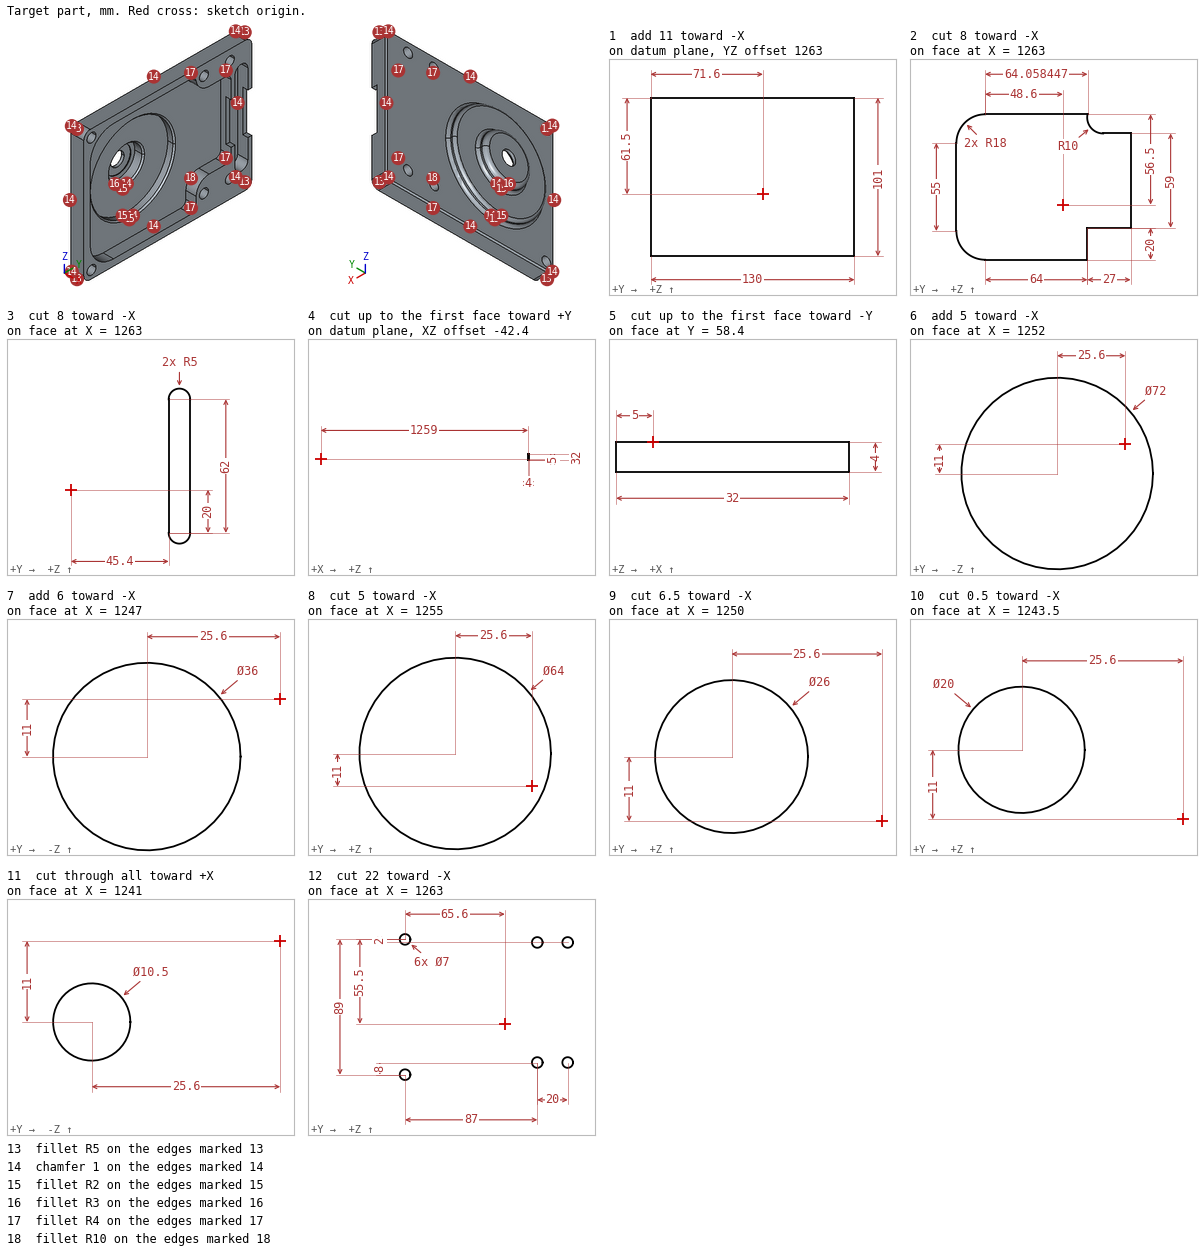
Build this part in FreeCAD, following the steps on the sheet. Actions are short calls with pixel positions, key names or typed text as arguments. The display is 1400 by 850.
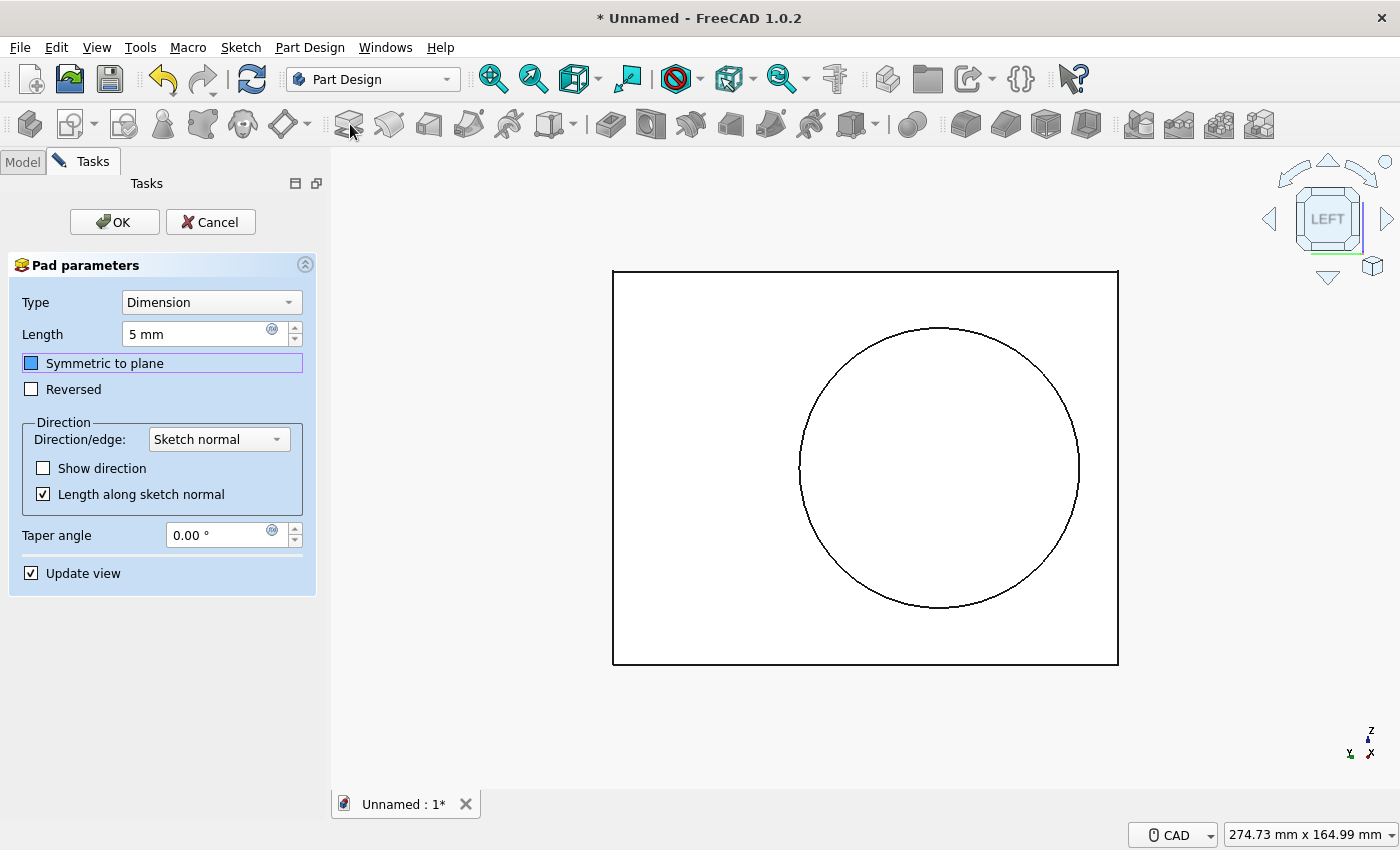
click(115, 222)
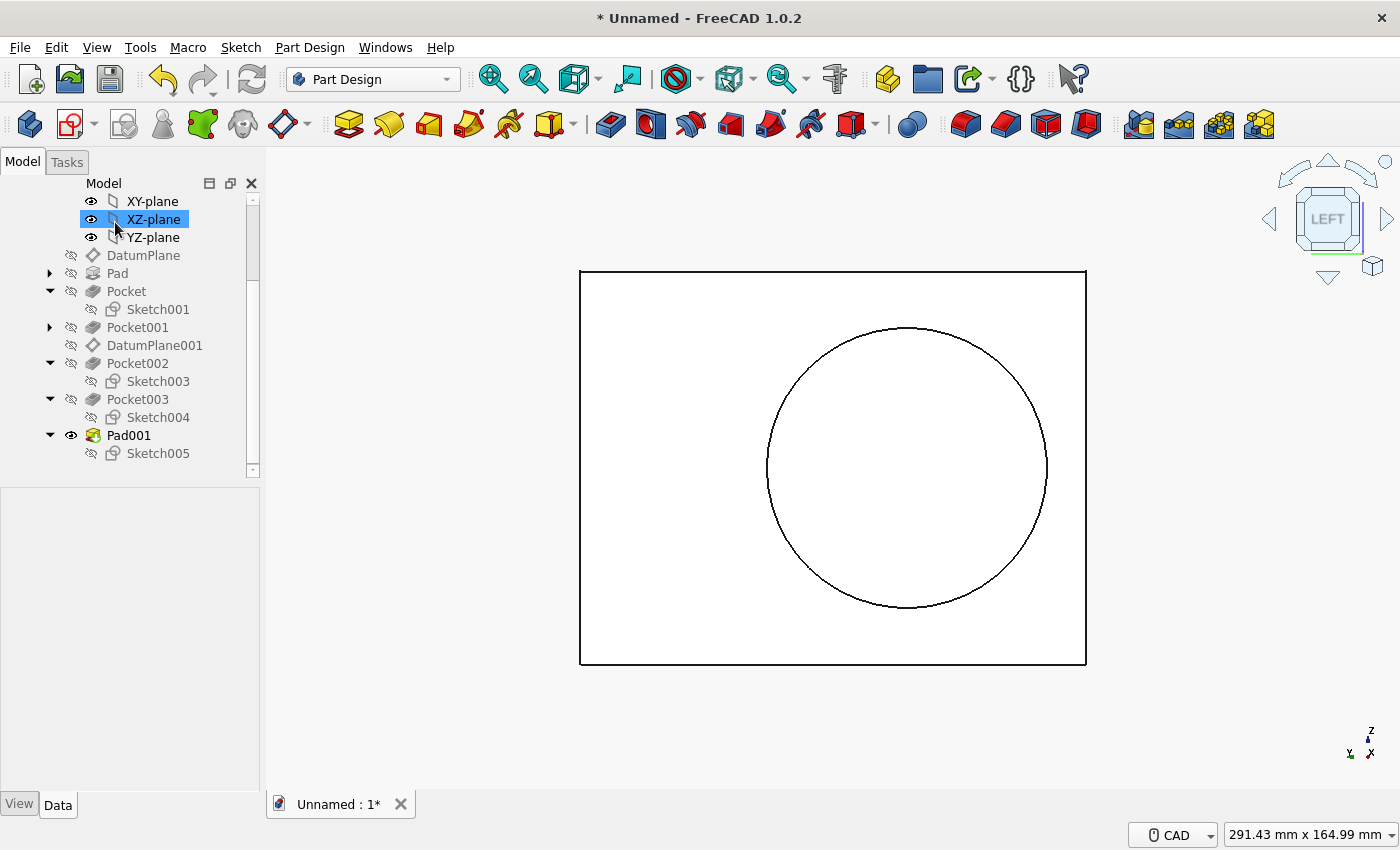
click(907, 467)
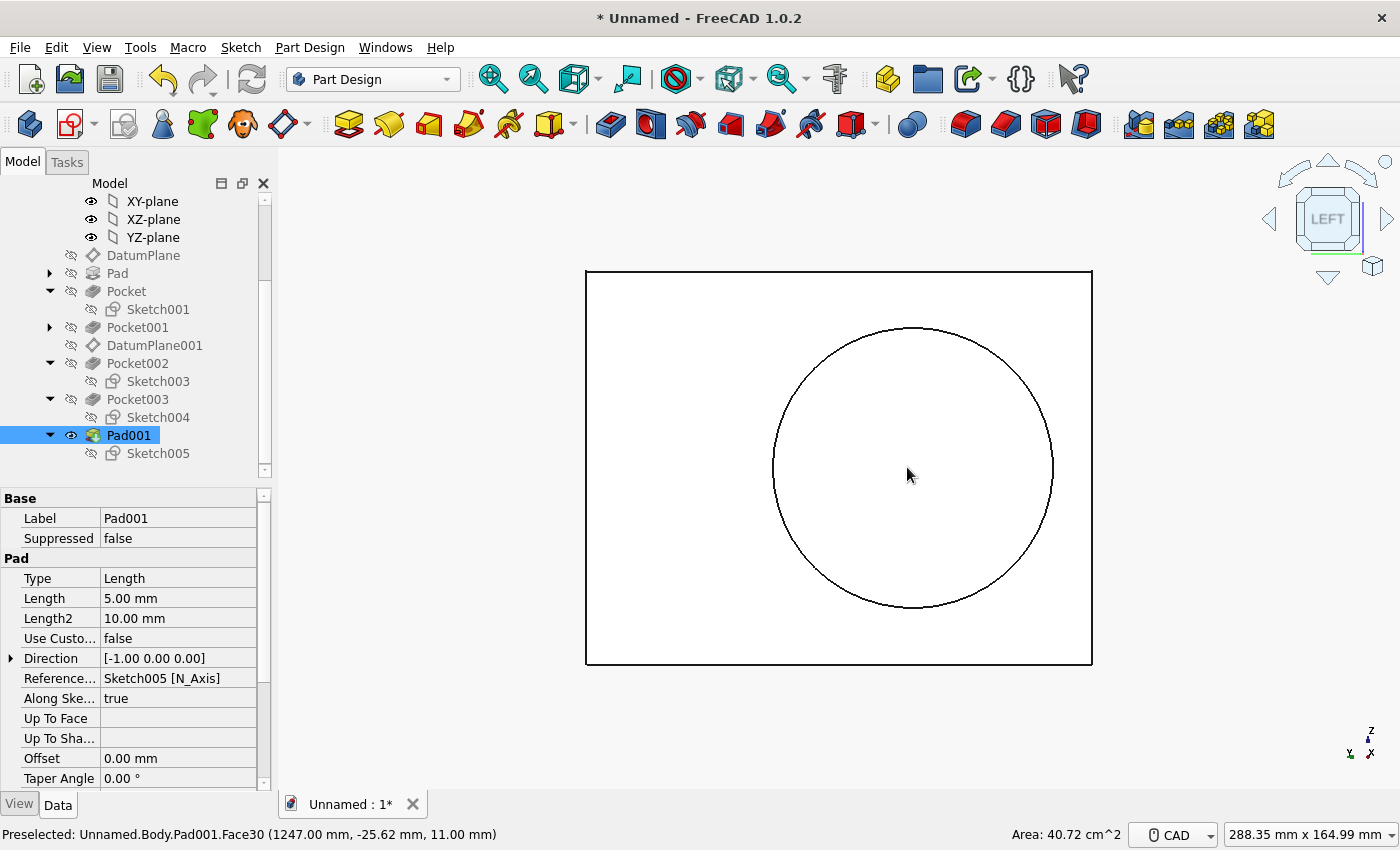
click(70, 124)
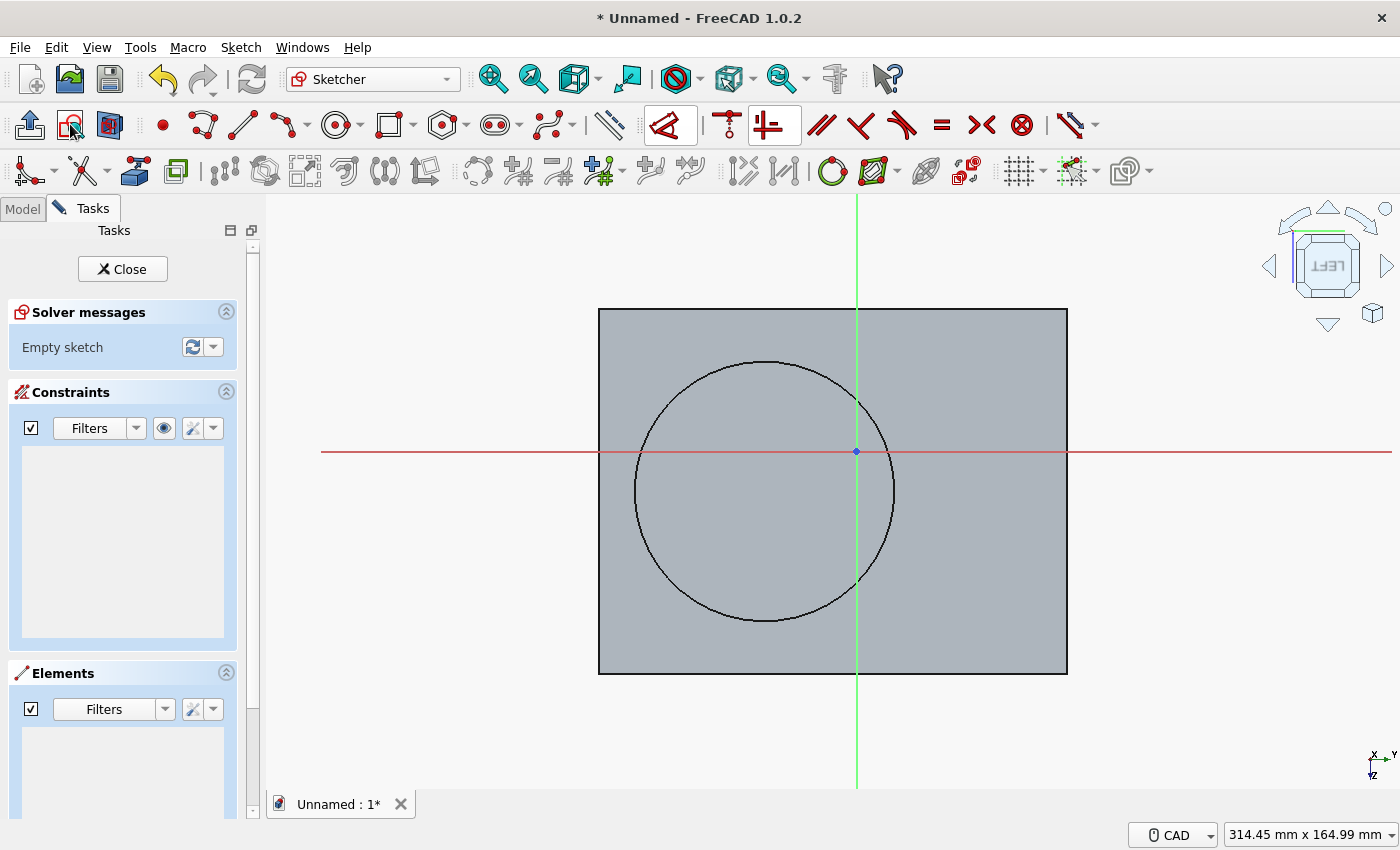
scroll(786, 491, up, 5)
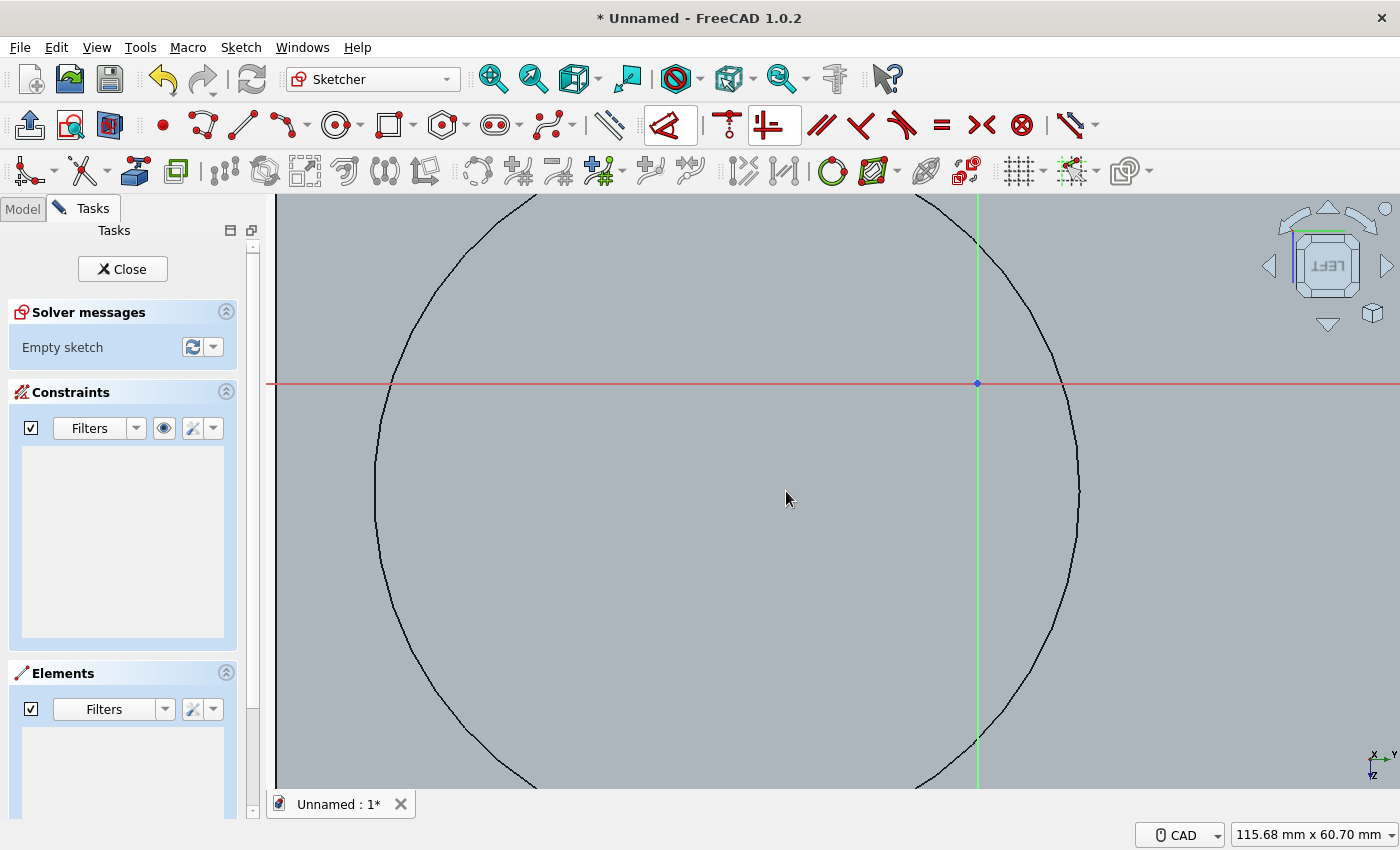
key(g)
key(c)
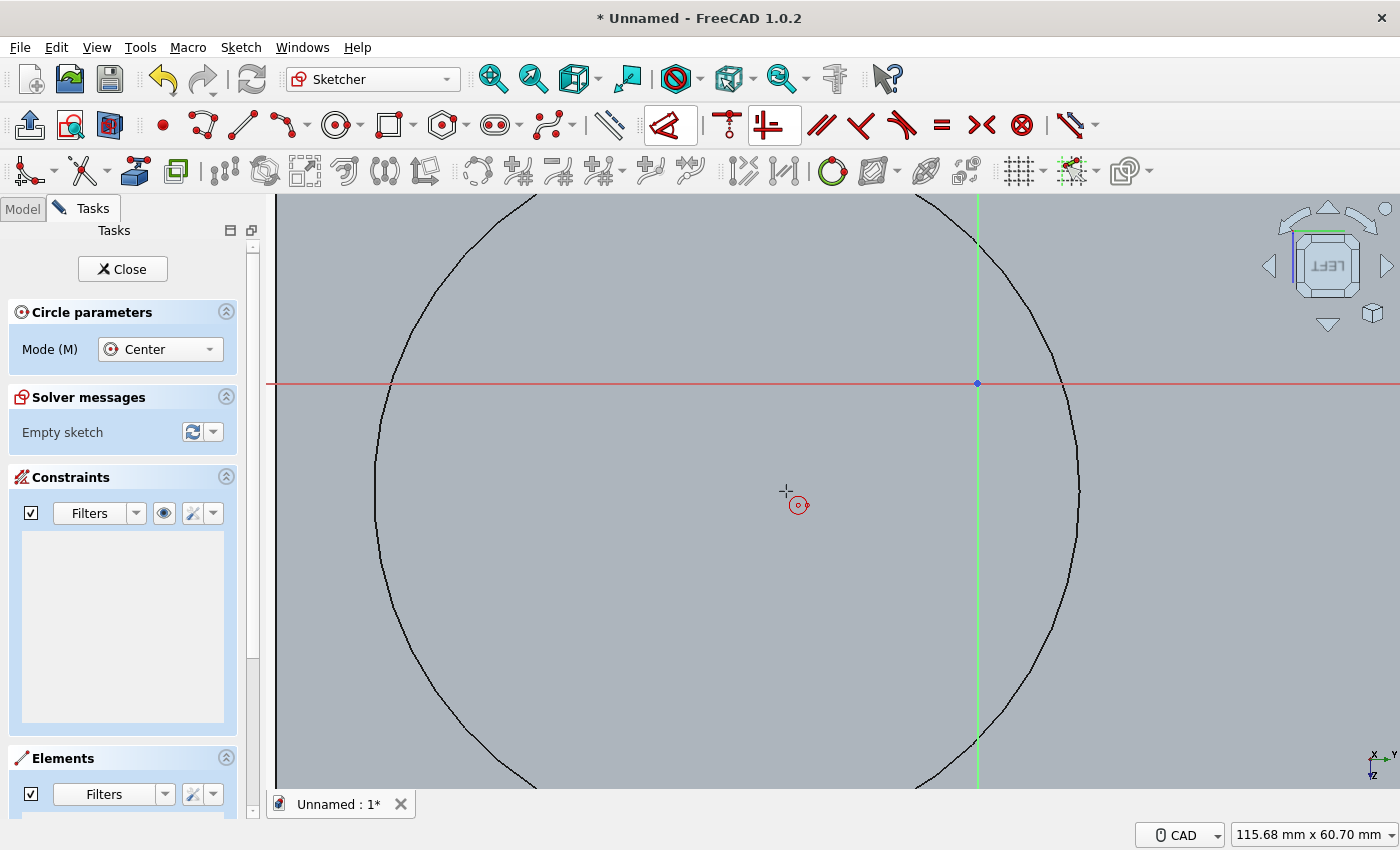
click(727, 491)
move(851, 367)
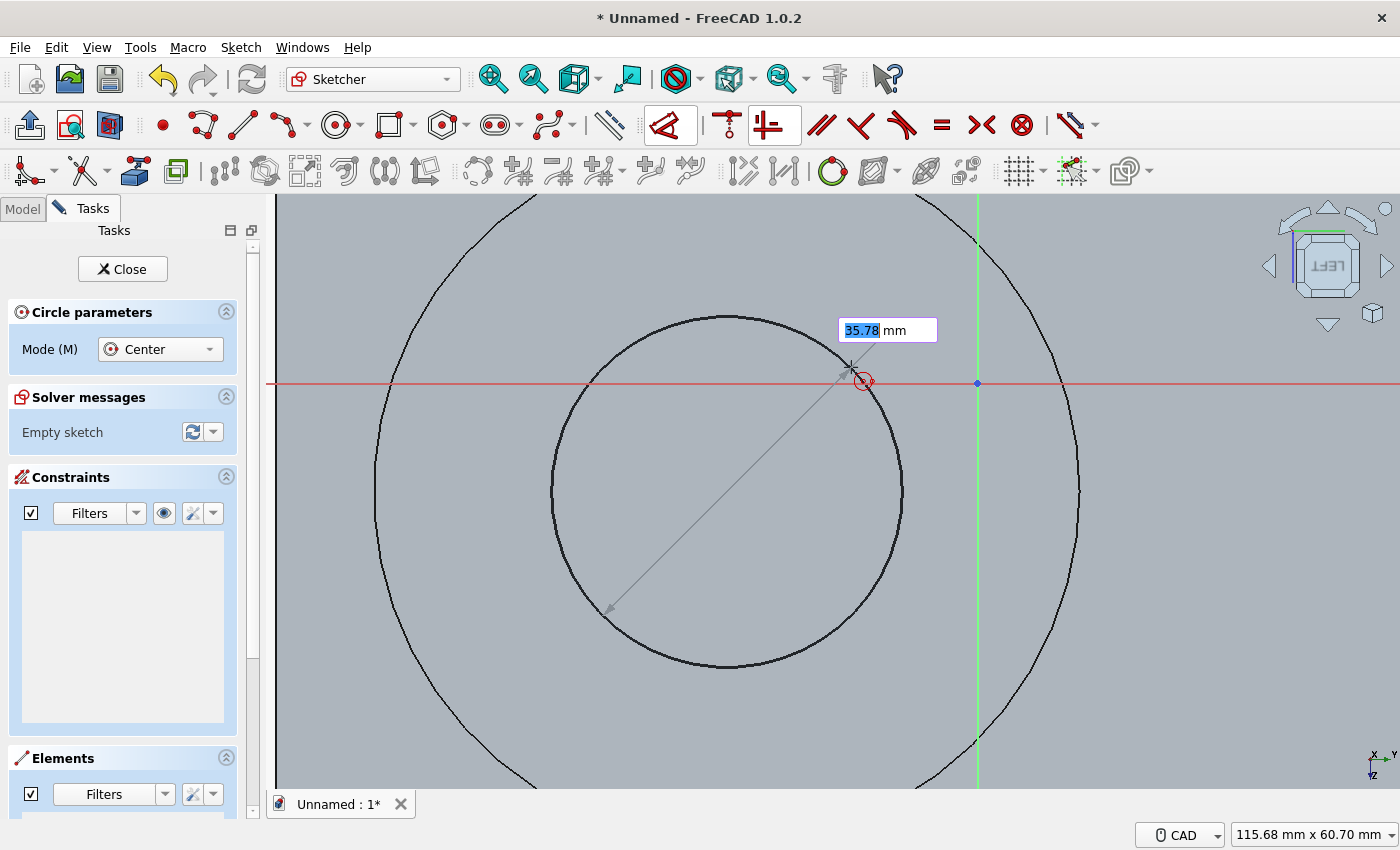
text(36)
key(Return)
key(Escape)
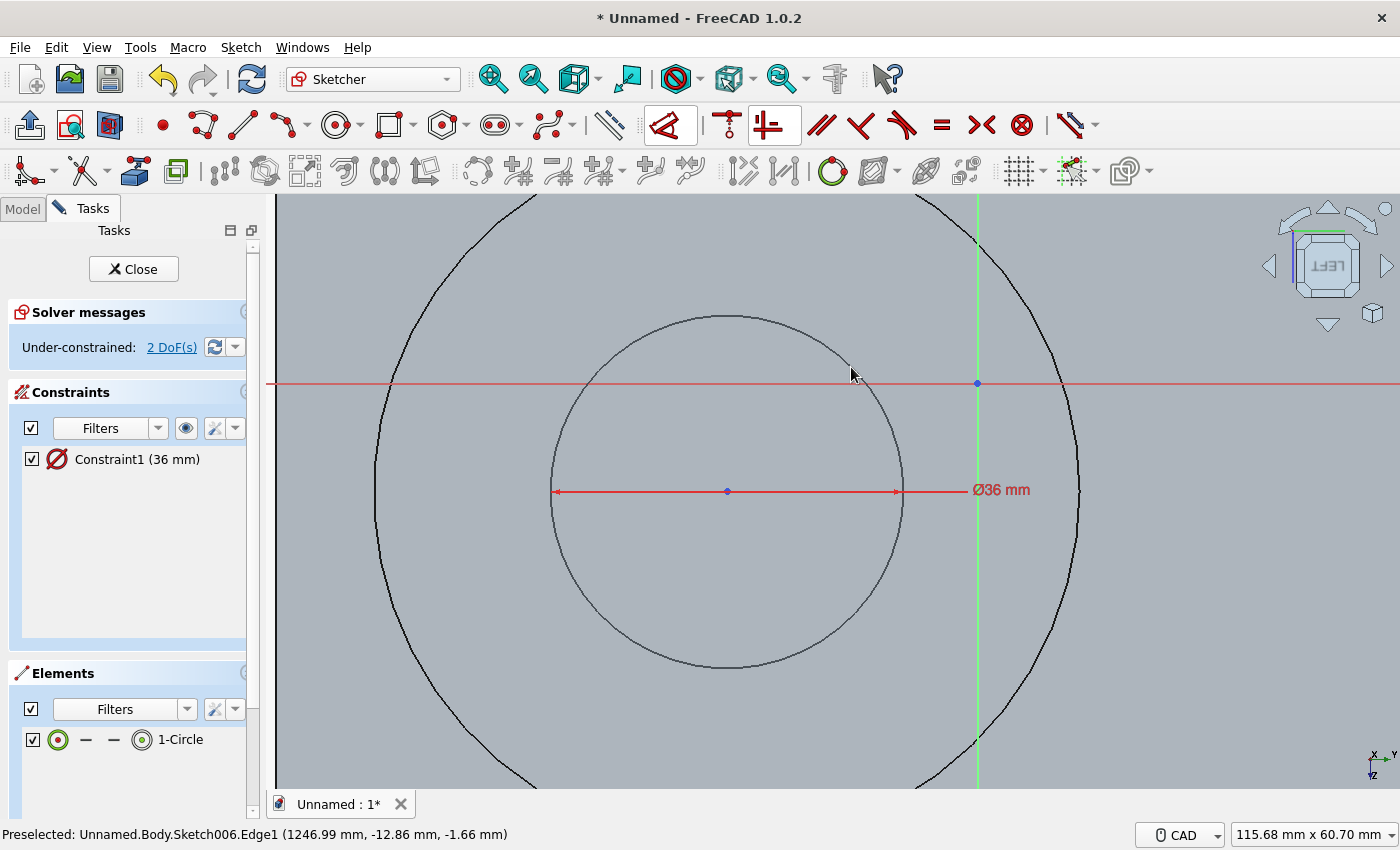
click(727, 492)